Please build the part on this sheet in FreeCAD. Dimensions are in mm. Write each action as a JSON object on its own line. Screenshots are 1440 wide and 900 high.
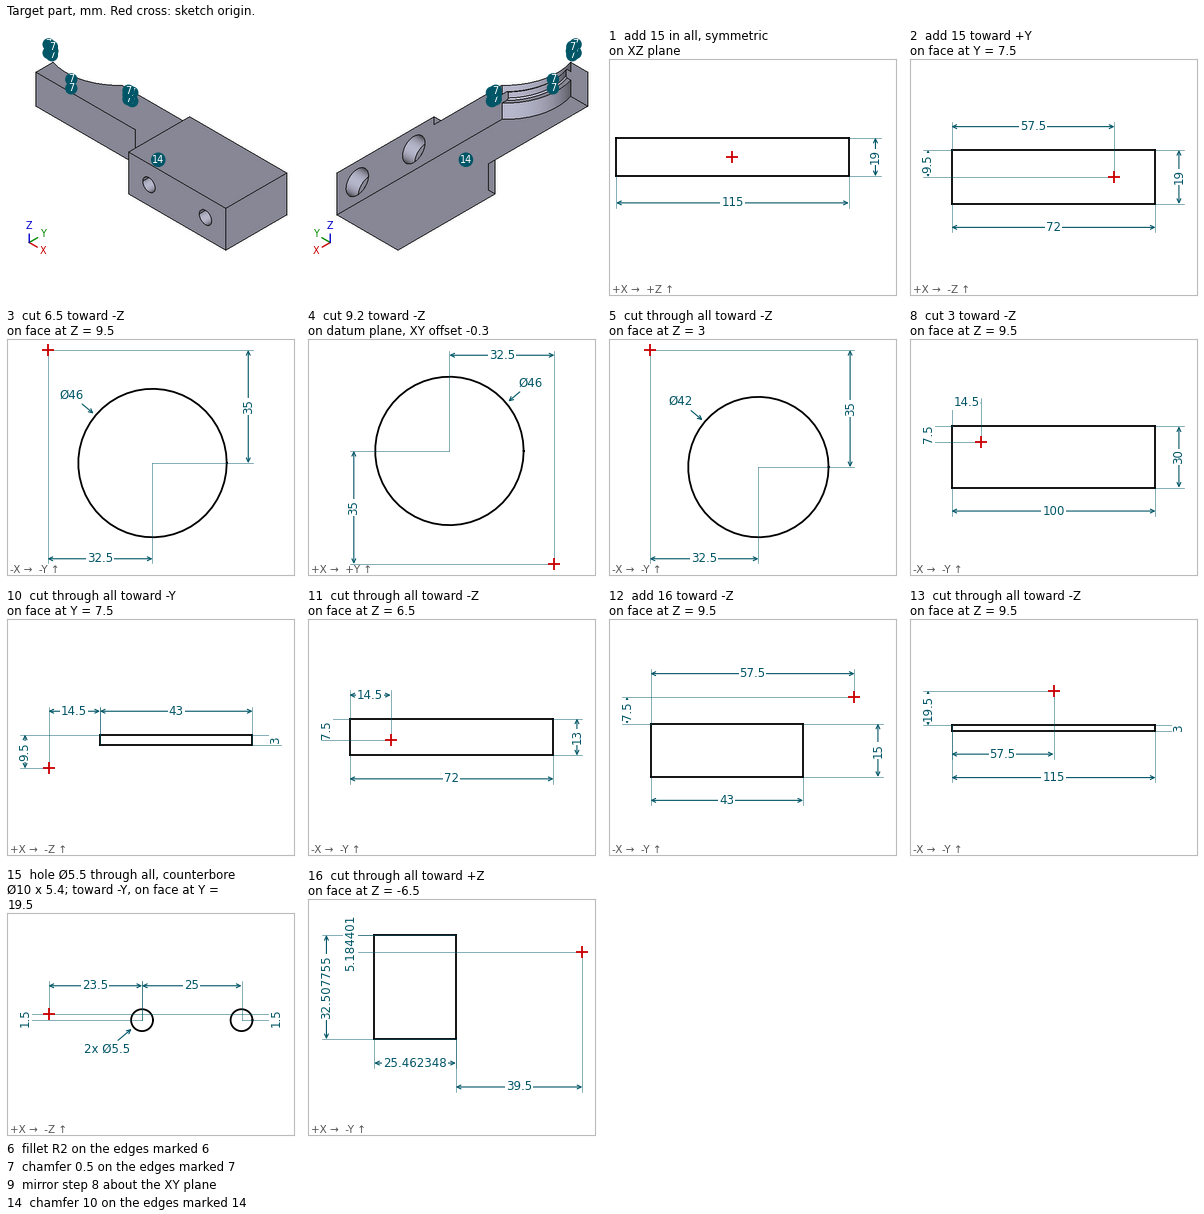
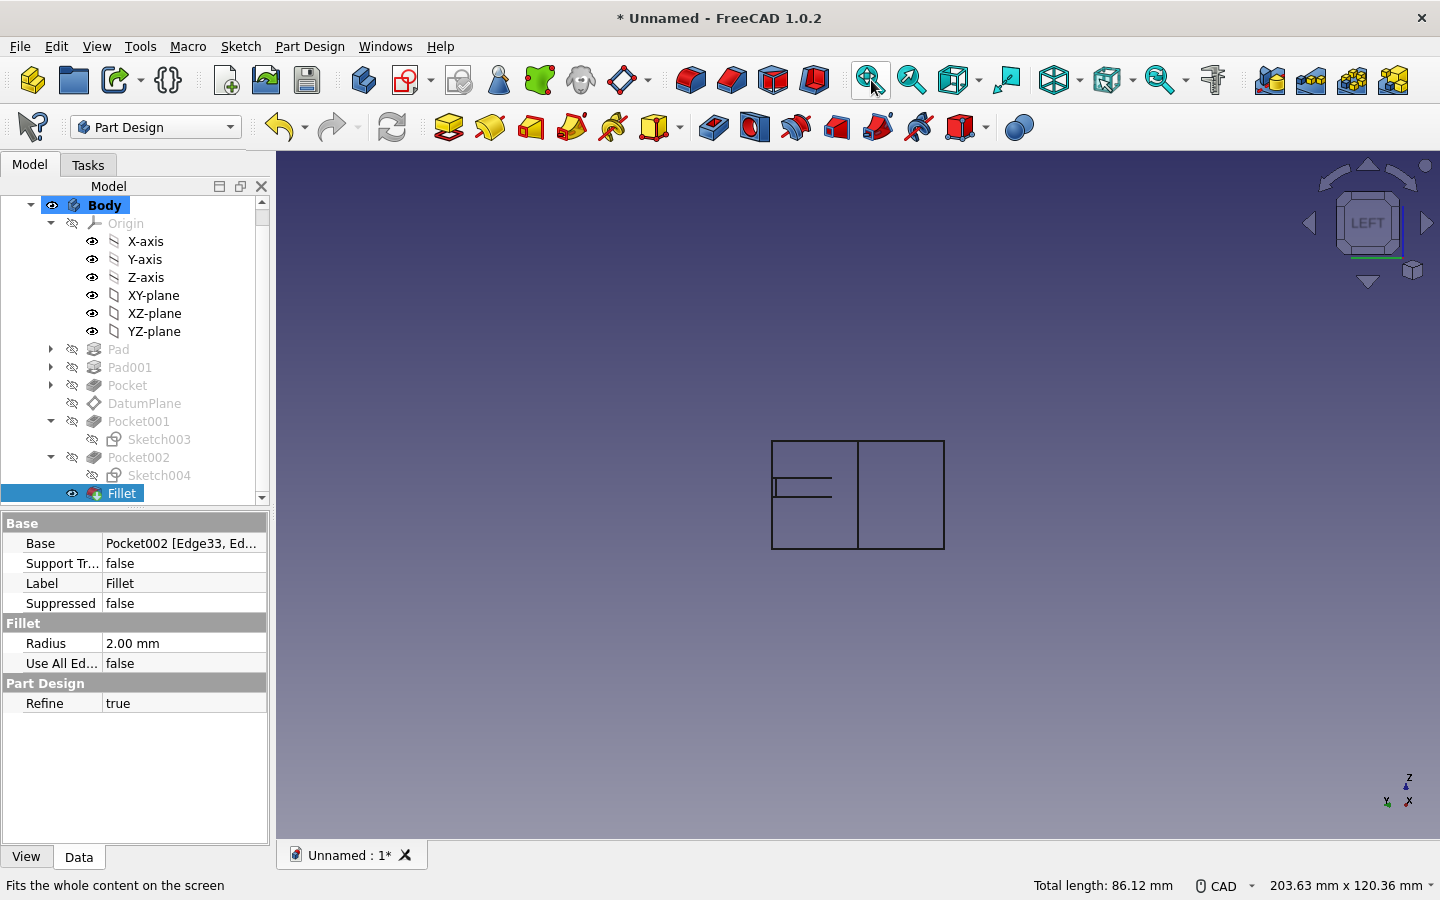
{"action": "key", "text": "0"}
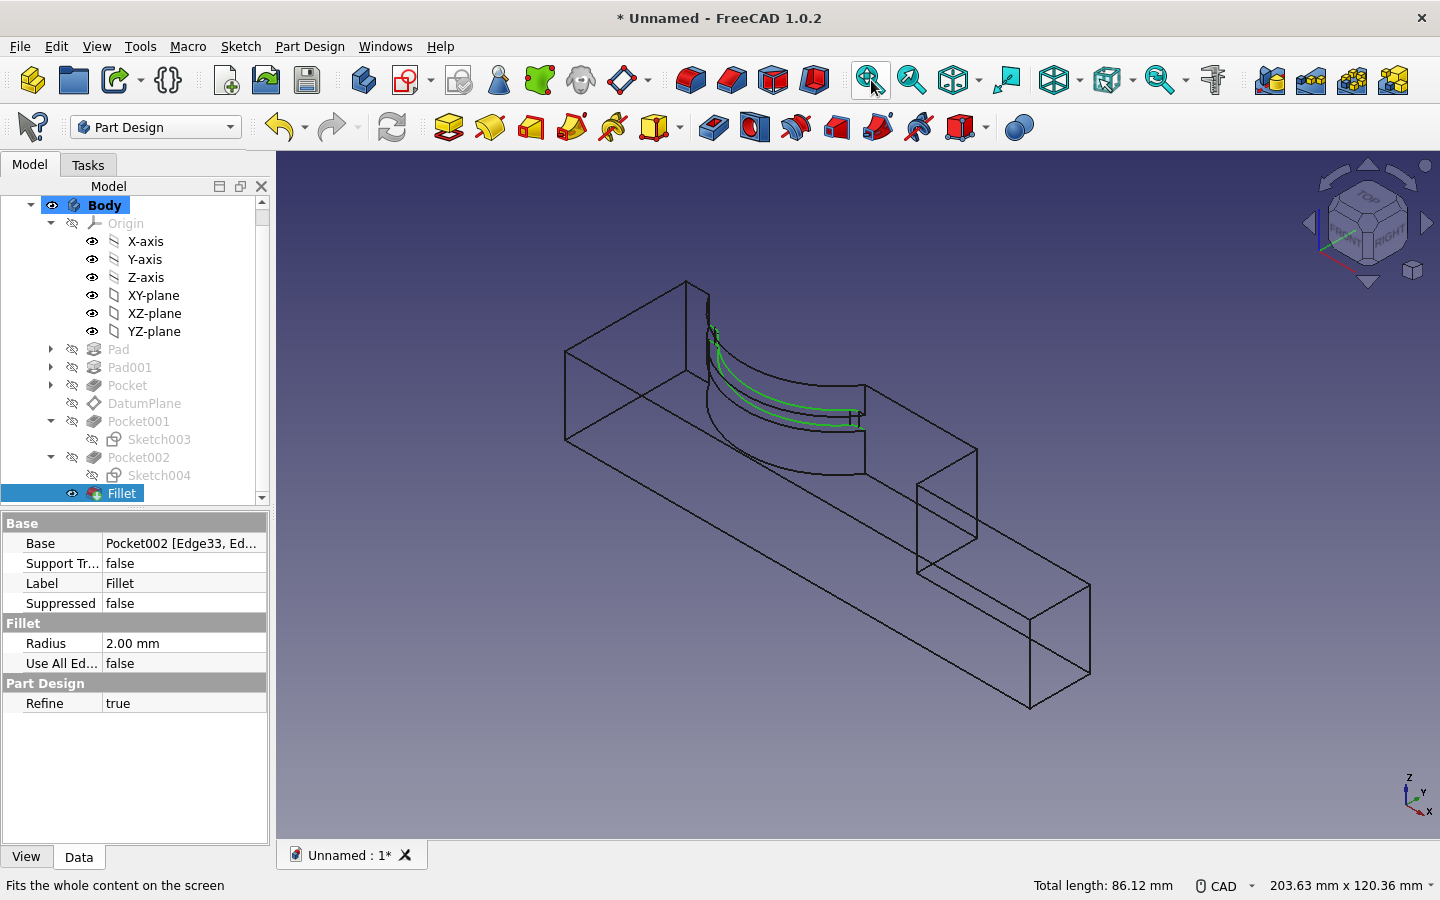
{"action": "scroll", "coordinate": [862, 413], "scroll_direction": "up", "scroll_amount": 8}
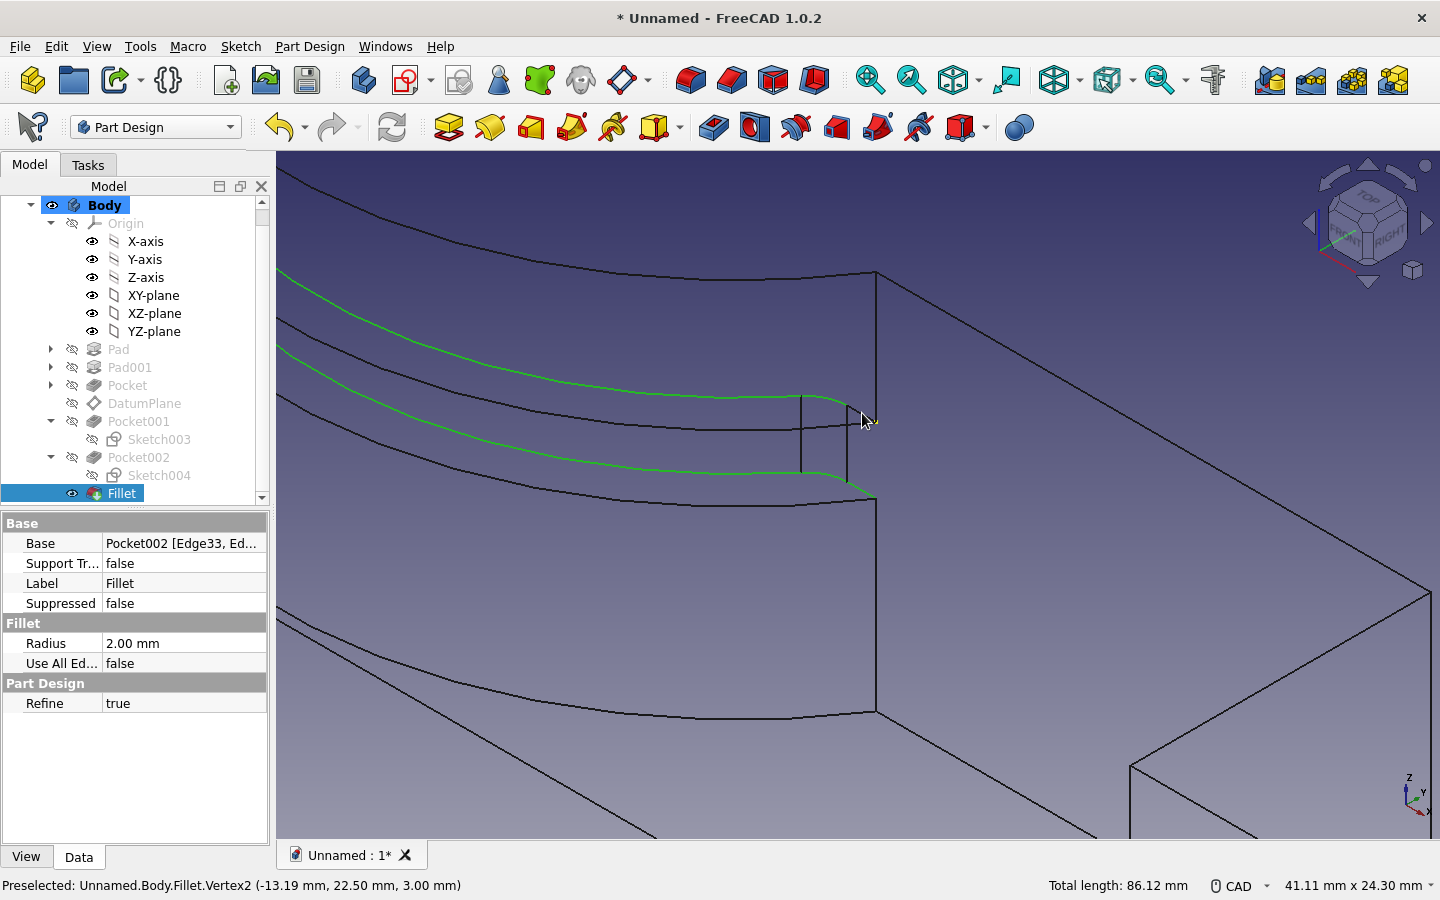
{"action": "left_click", "coordinate": [862, 413], "text": "ctrl"}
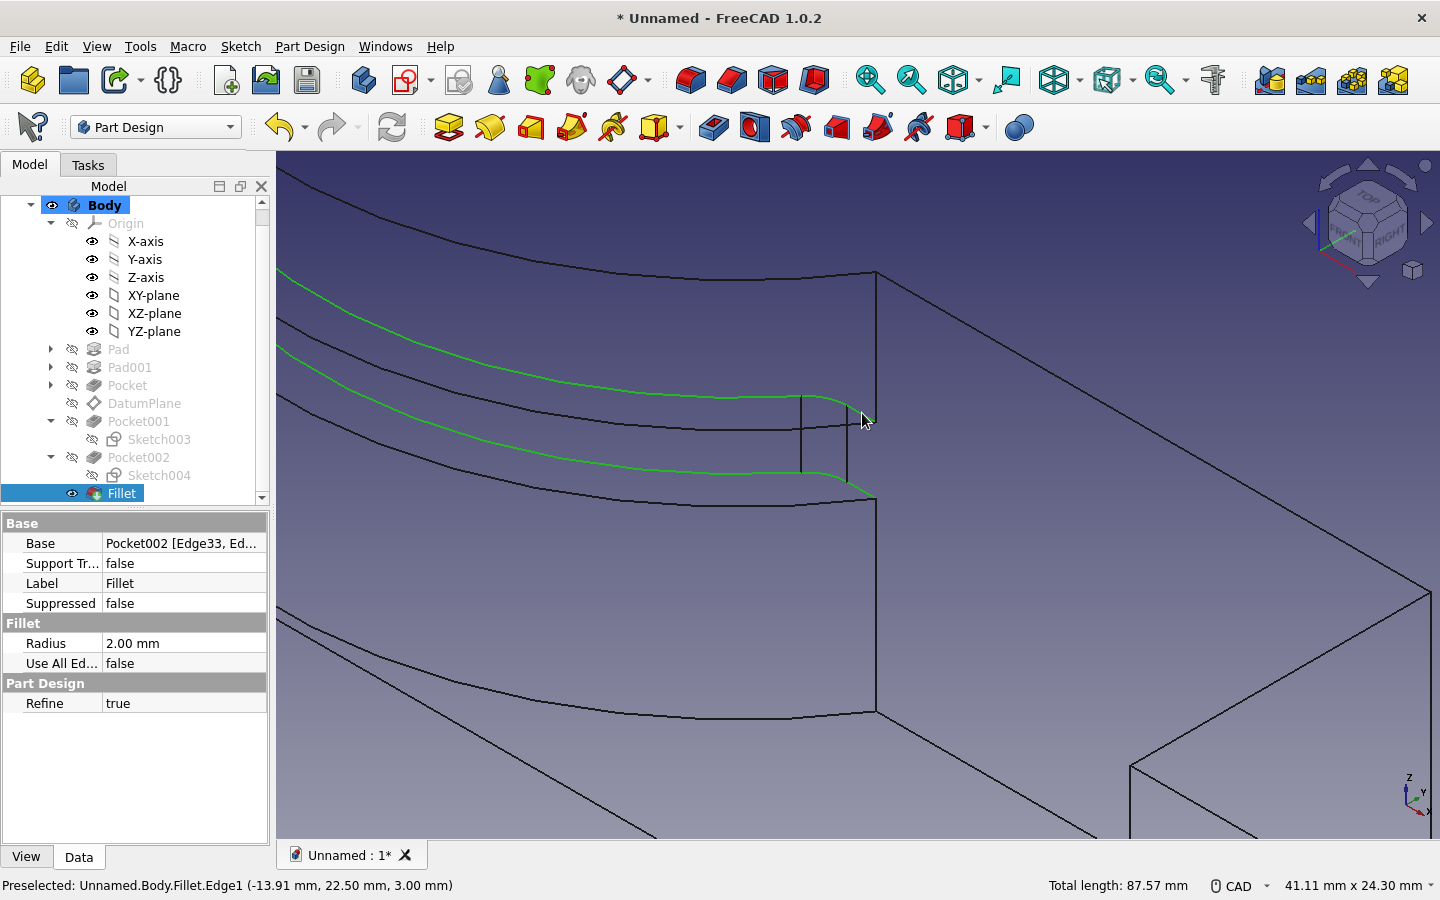
{"action": "key", "text": "v 1"}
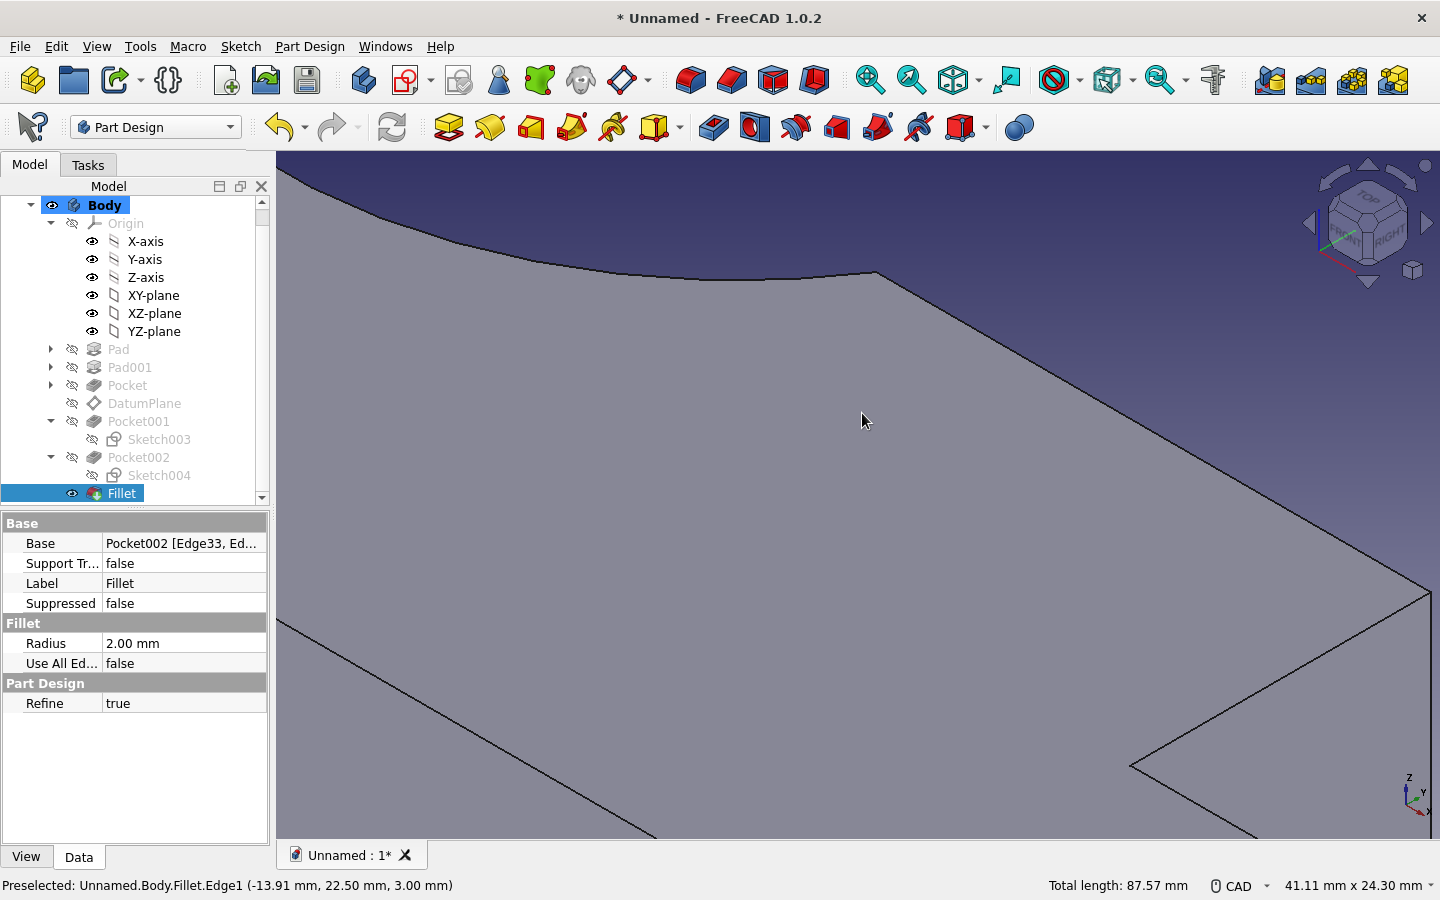
{"action": "left_click", "coordinate": [732, 80]}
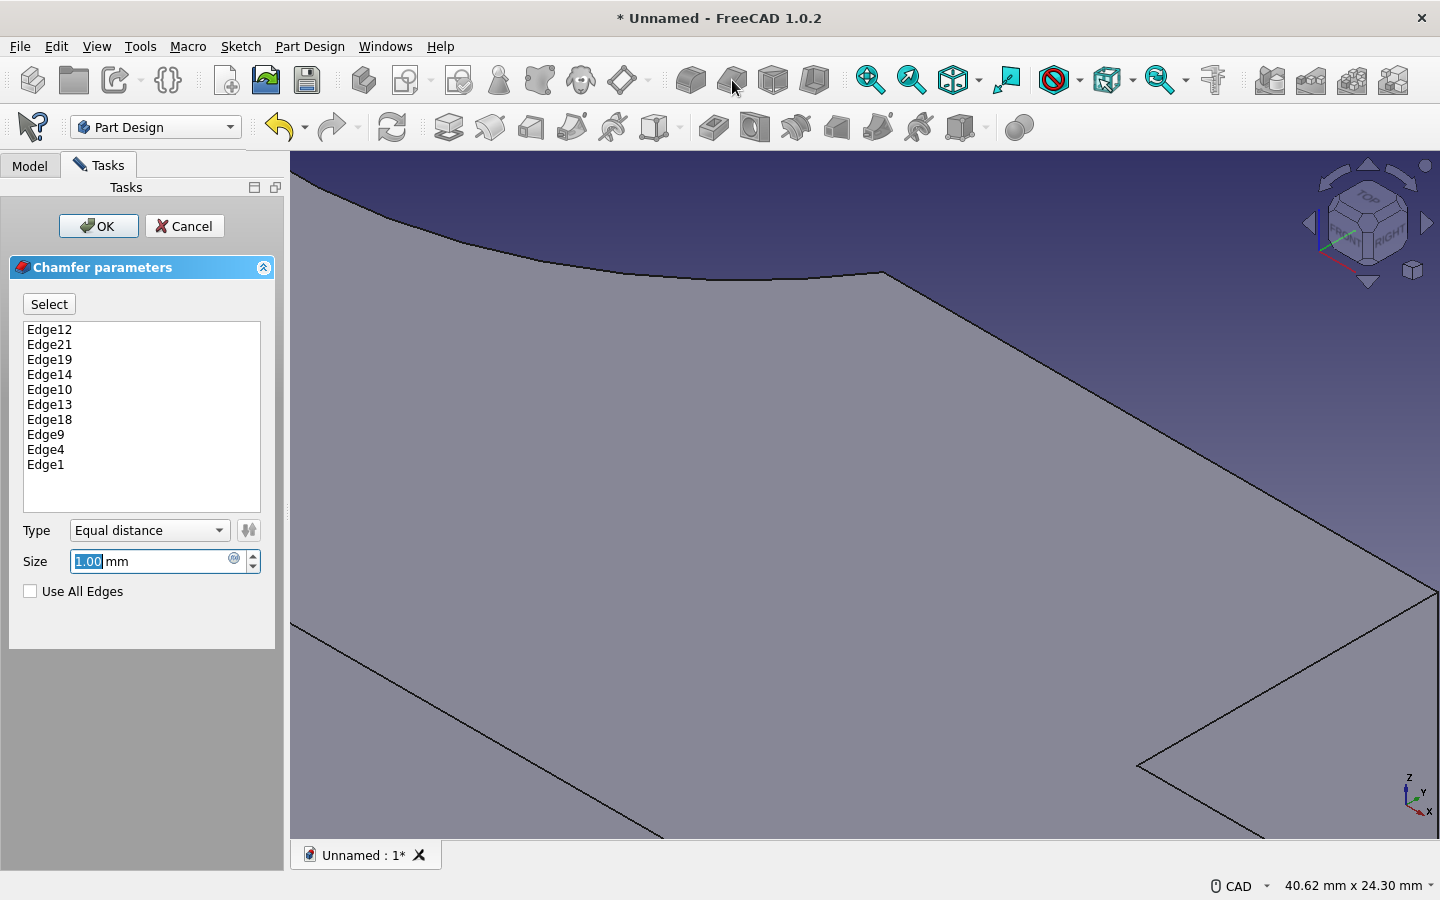
{"action": "type", "text": "0.5"}
{"action": "key", "text": "Tab"}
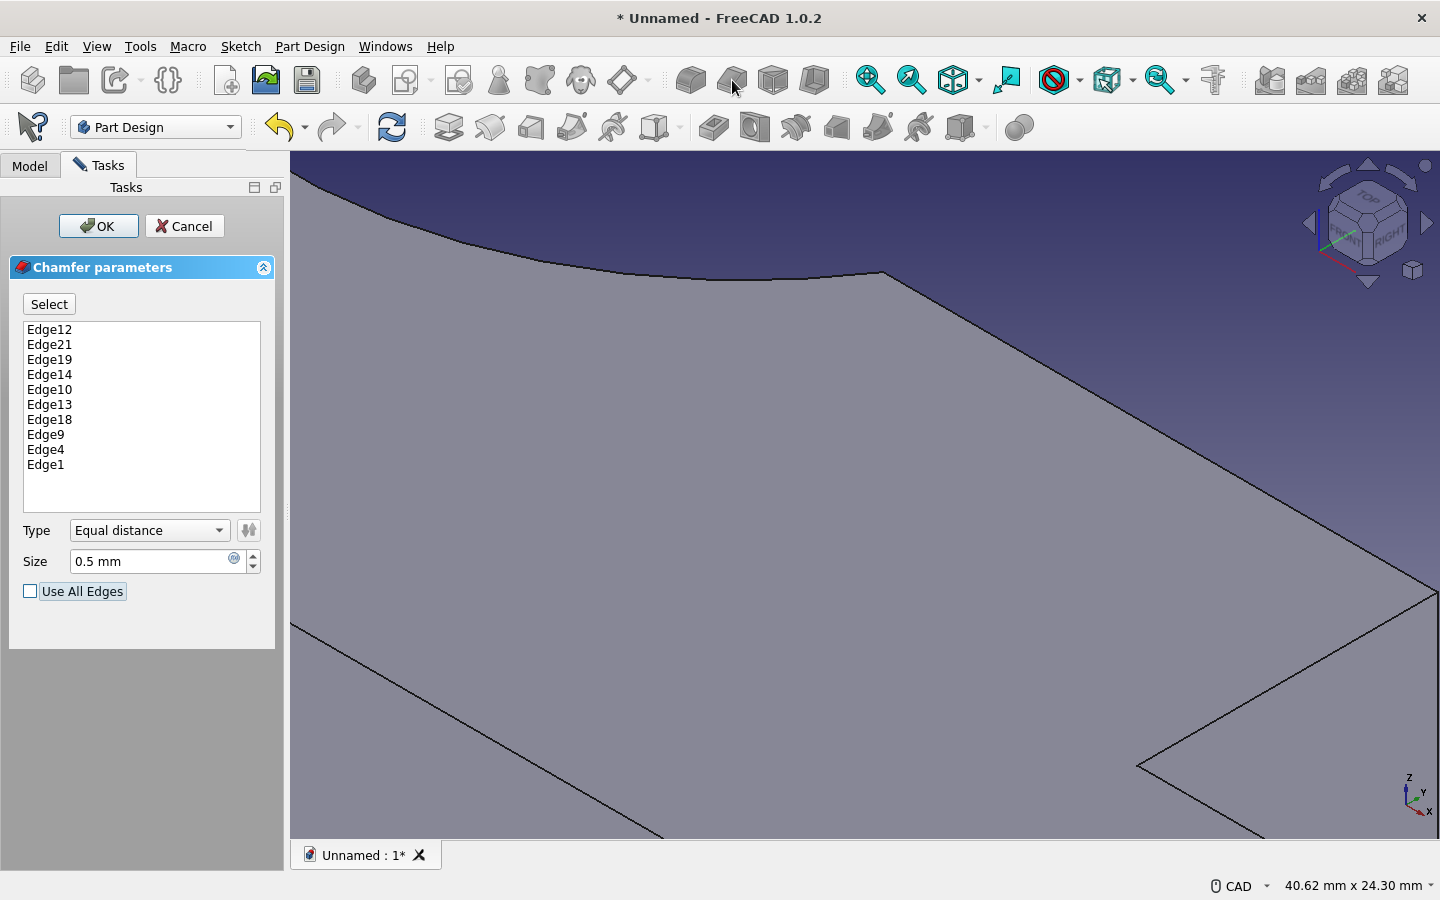
{"action": "left_click", "coordinate": [99, 226]}